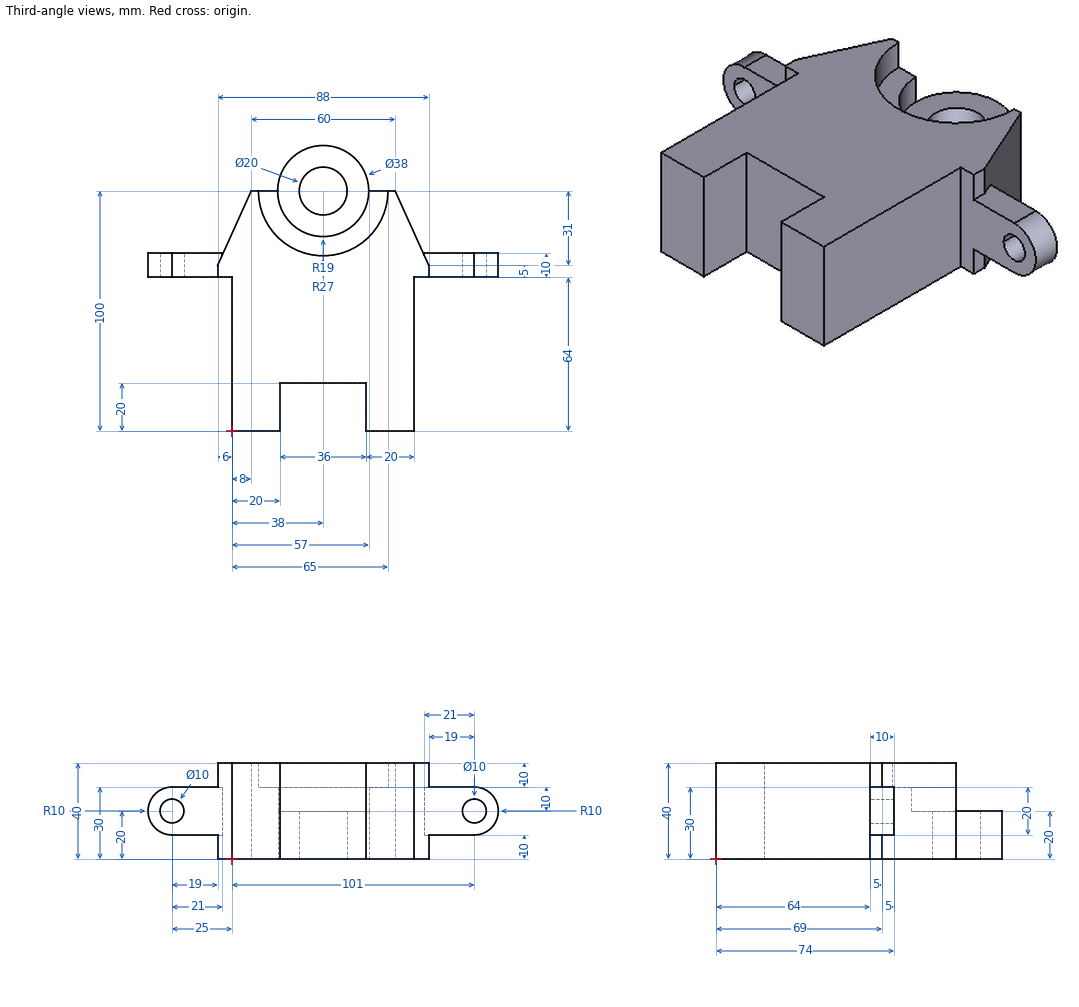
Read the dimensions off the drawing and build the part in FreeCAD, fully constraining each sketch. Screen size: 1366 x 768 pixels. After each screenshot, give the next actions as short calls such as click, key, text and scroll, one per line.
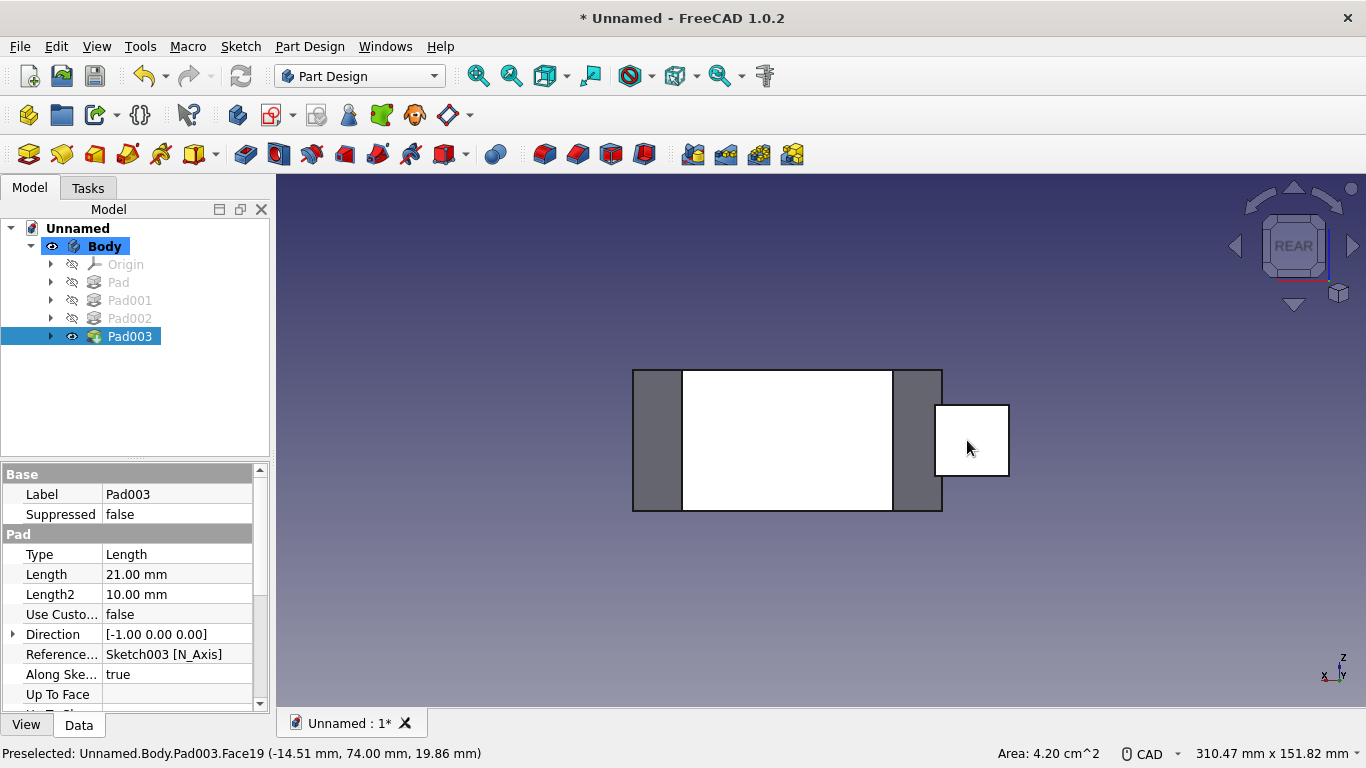
click(270, 116)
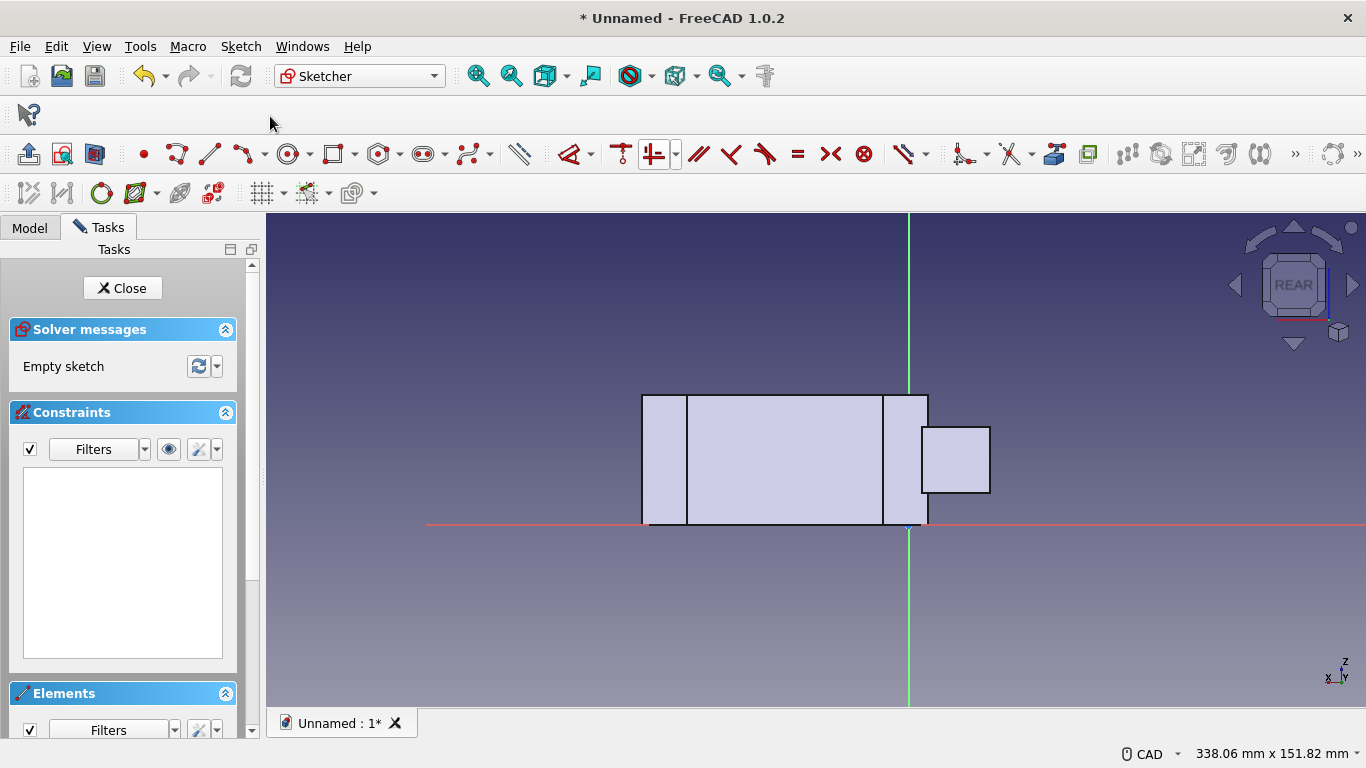
scroll(1060, 483, up, 6)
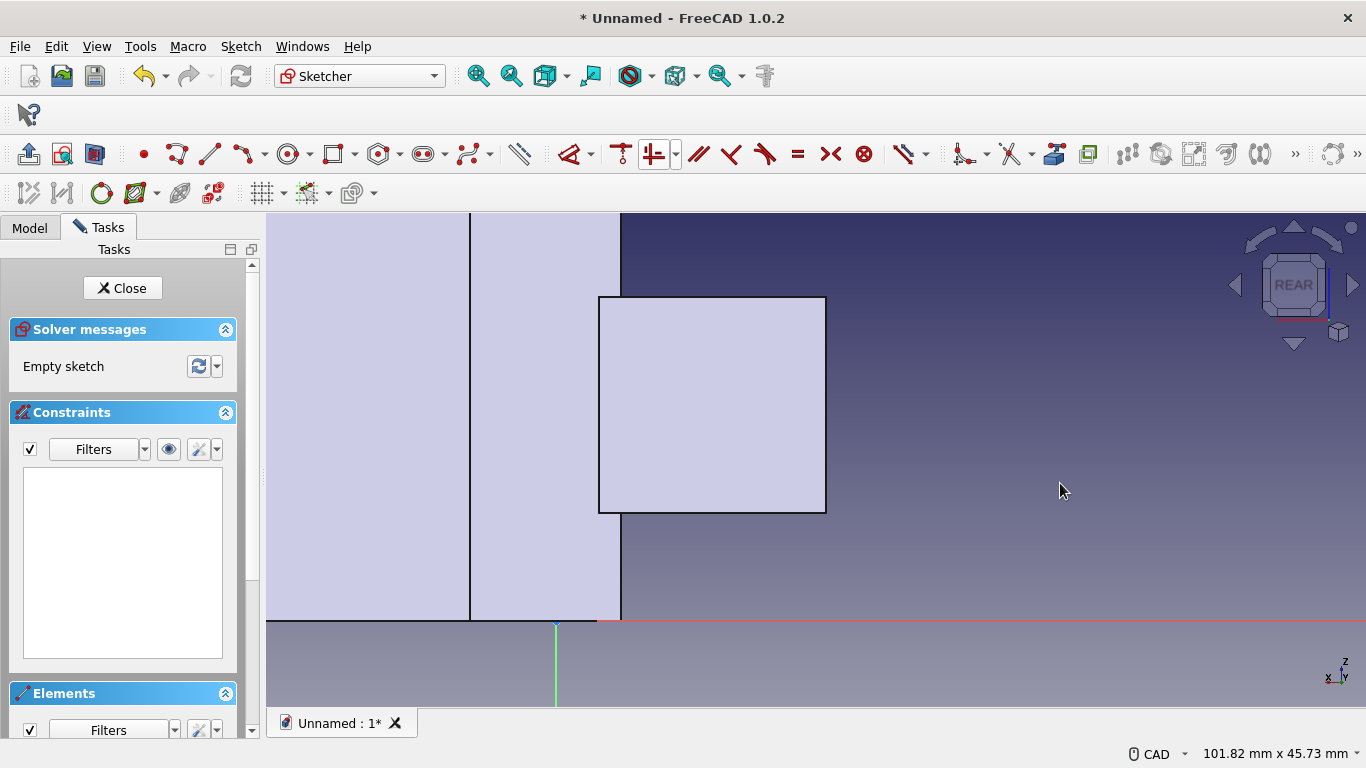
click(210, 154)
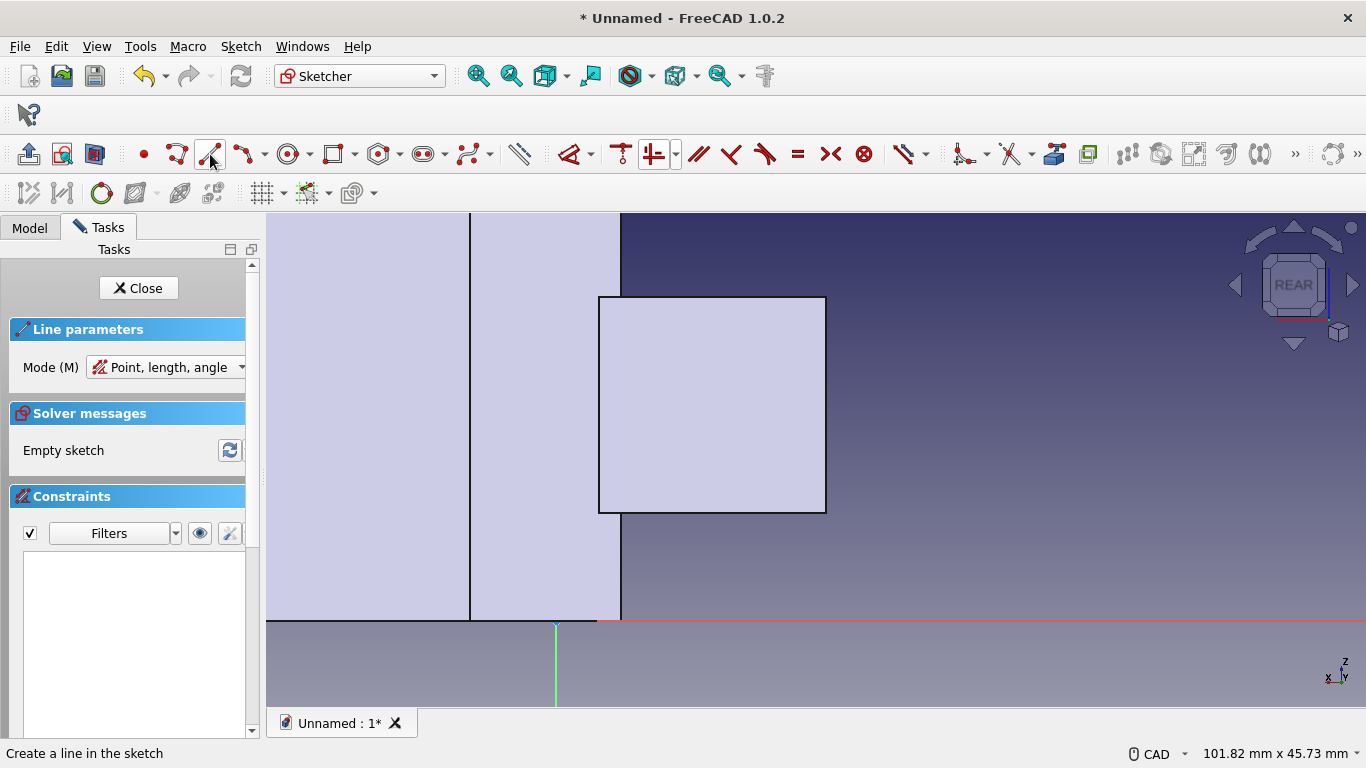
click(826, 297)
click(826, 513)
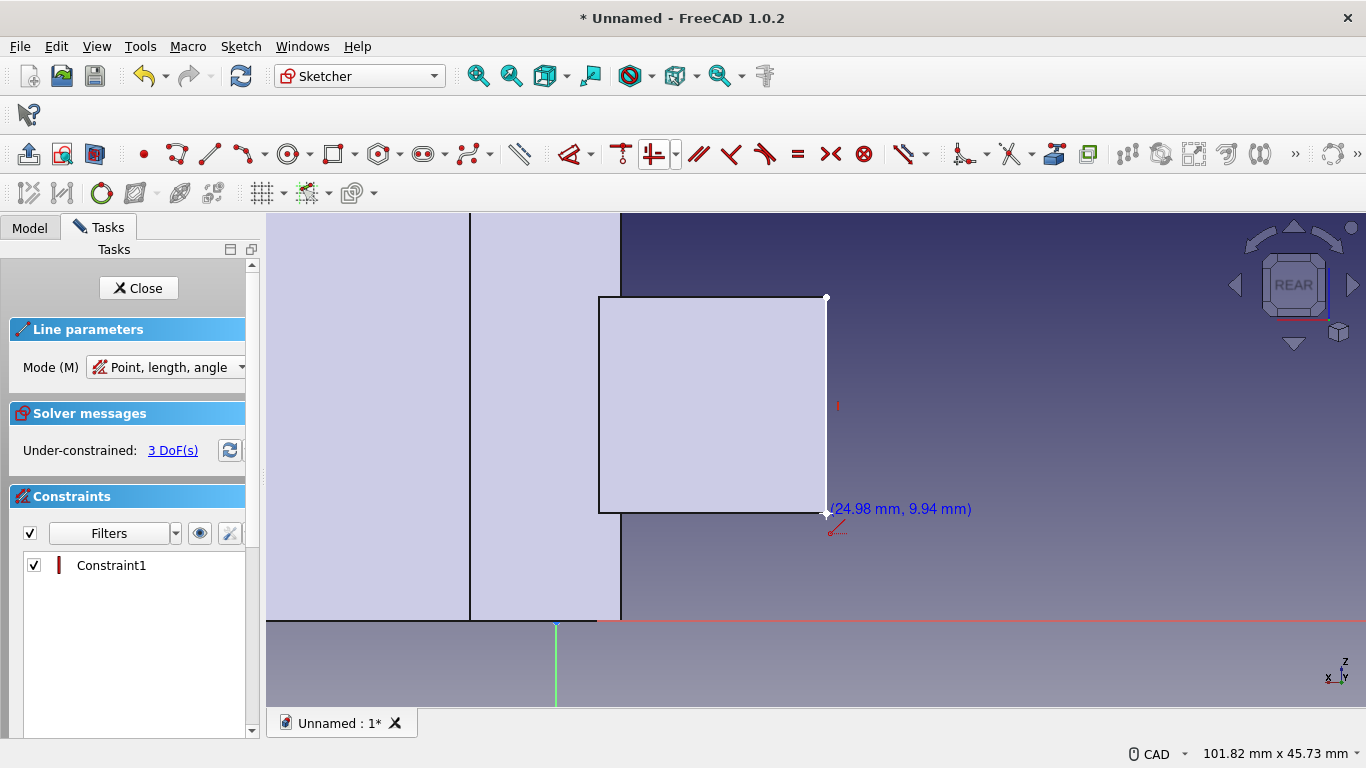
click(242, 154)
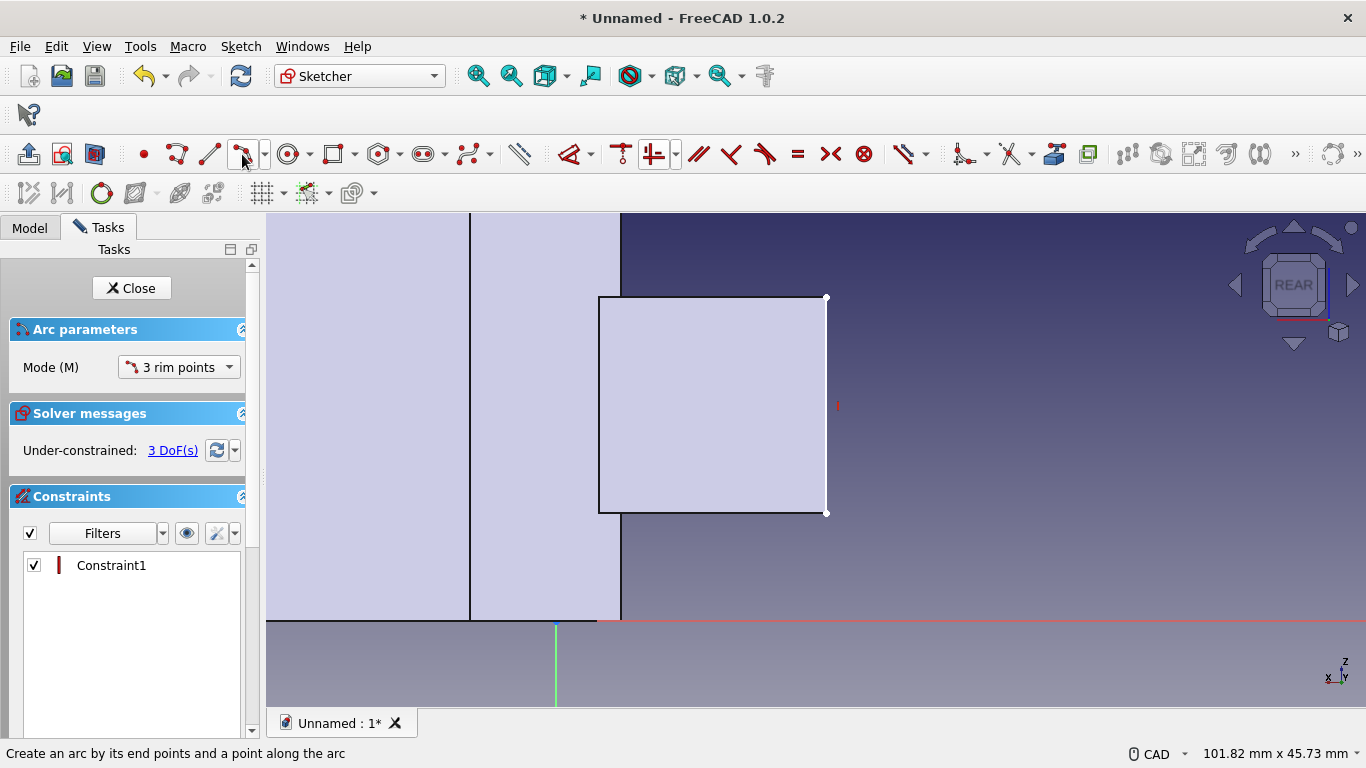
click(826, 514)
click(826, 298)
click(934, 405)
key(Escape)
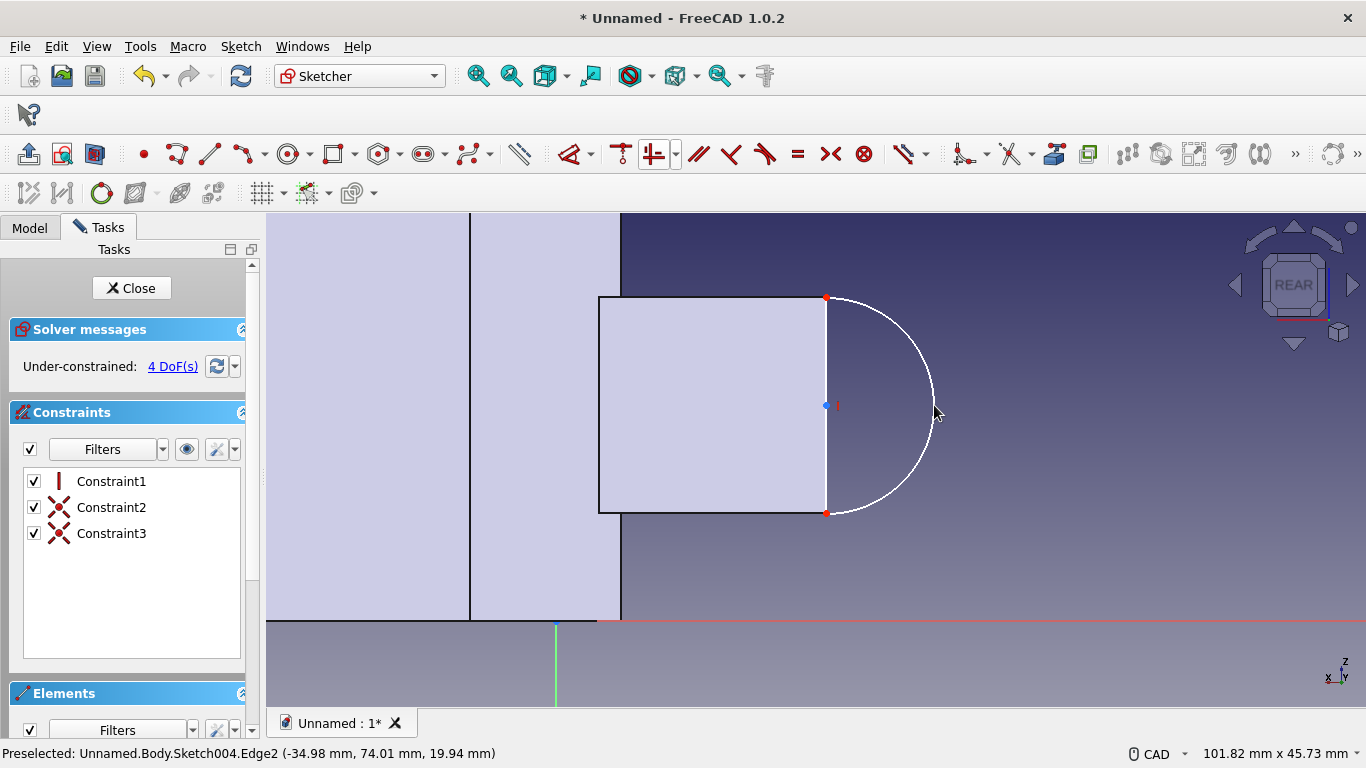
click(568, 154)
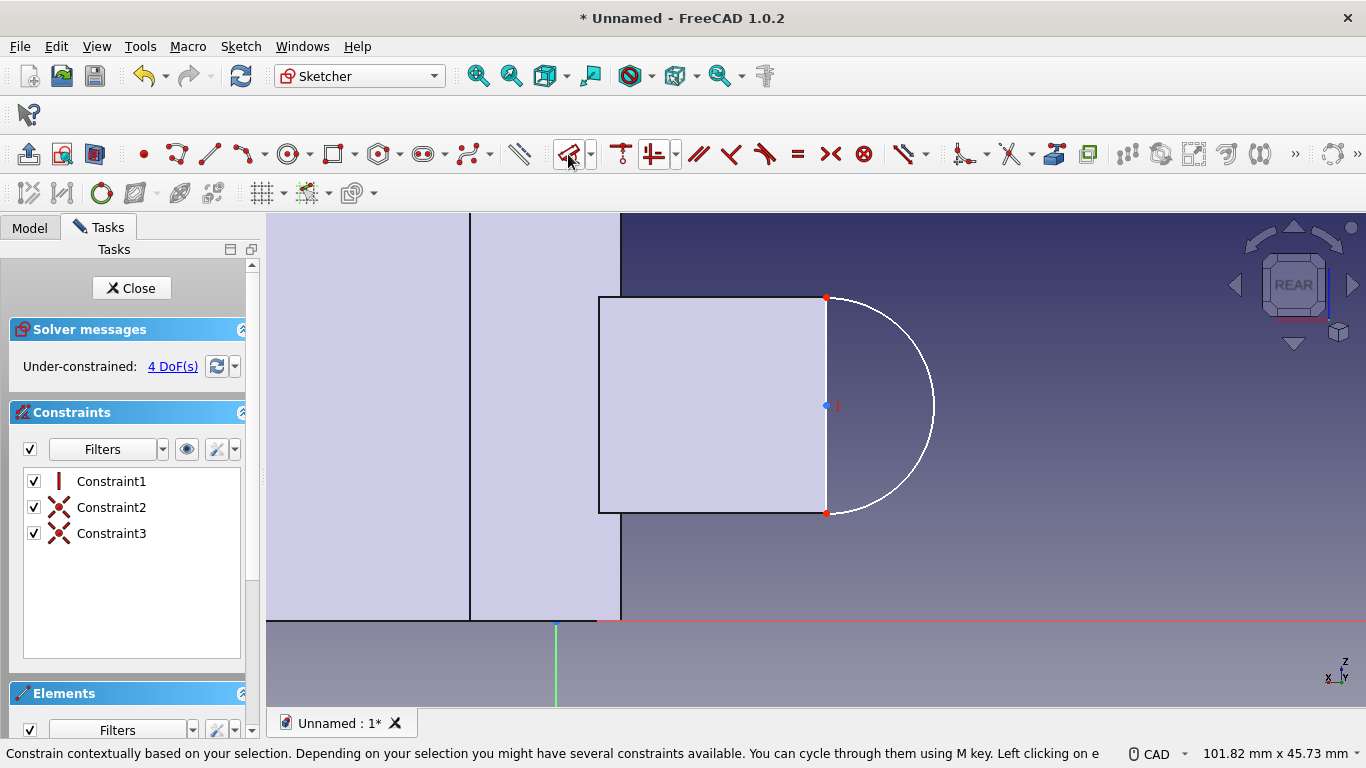
click(913, 469)
click(939, 488)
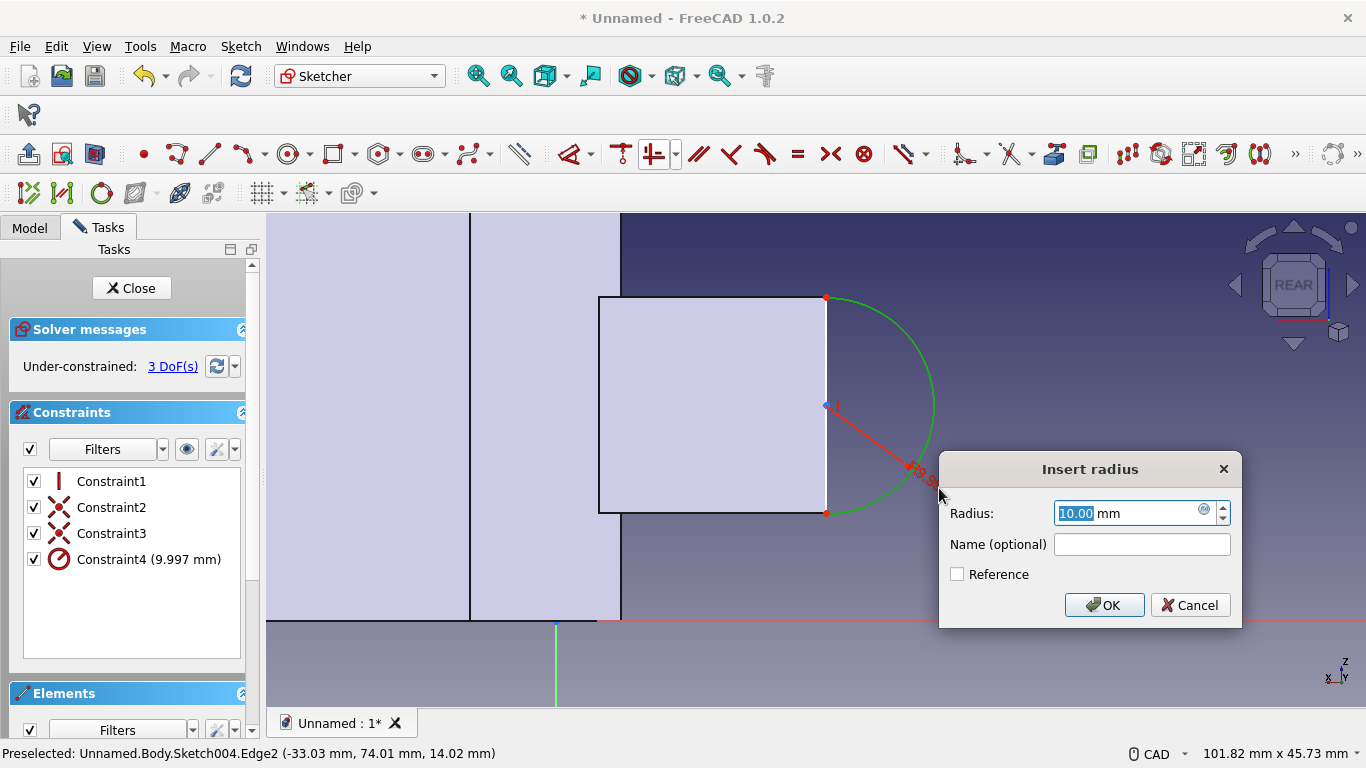
text(10)
key(Return)